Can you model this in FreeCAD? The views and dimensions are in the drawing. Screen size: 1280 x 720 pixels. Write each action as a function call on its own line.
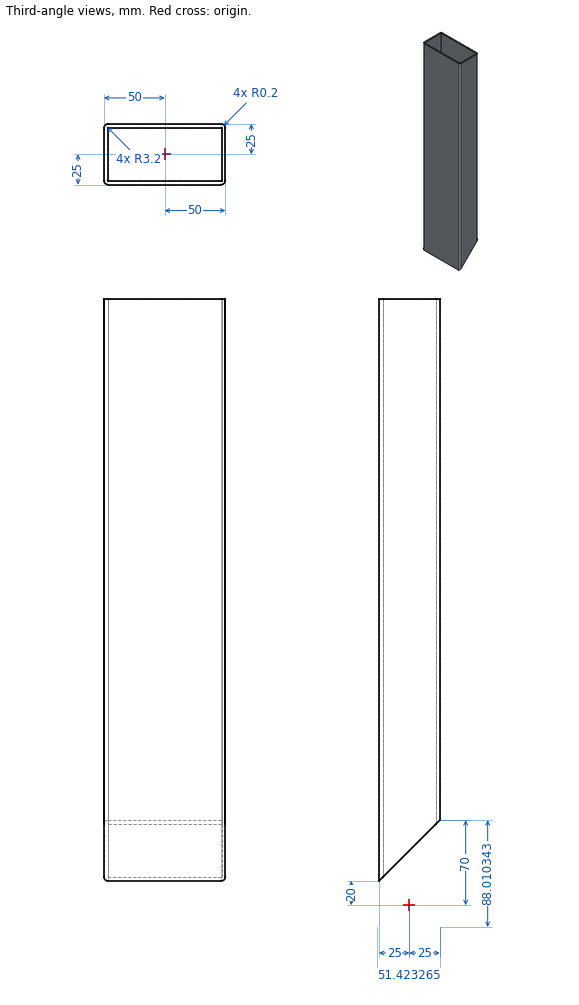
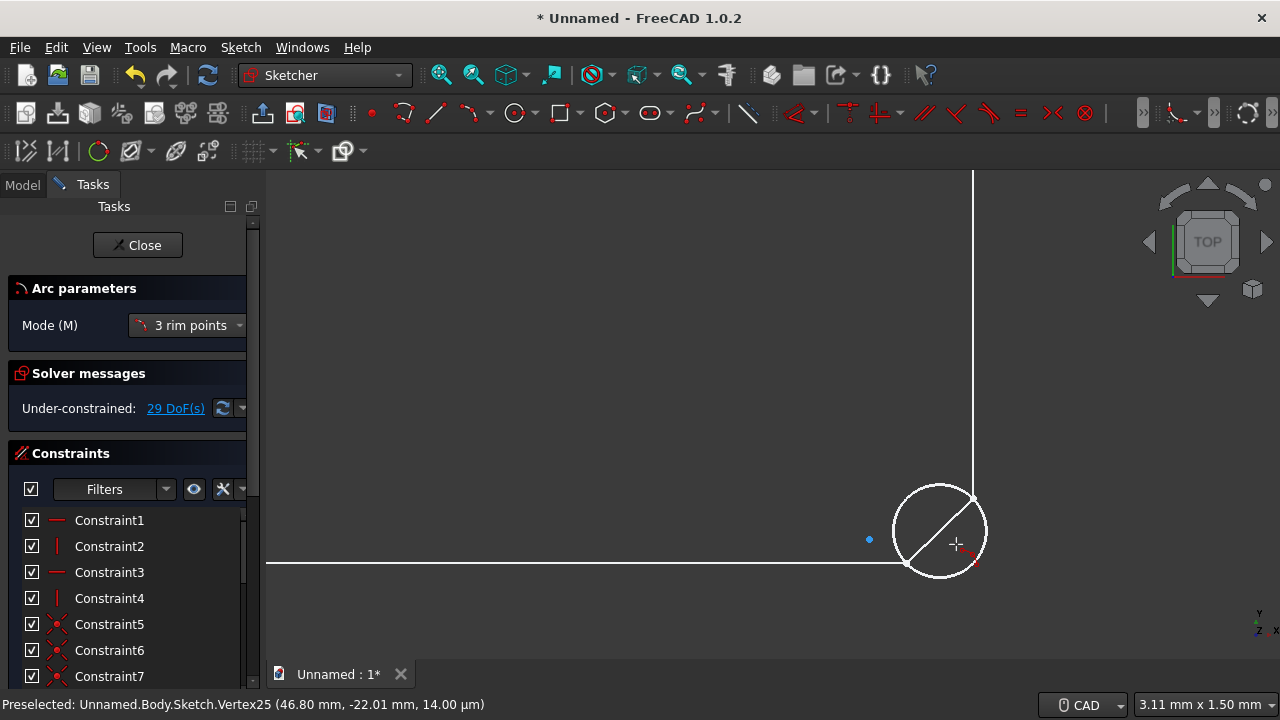
click(953, 540)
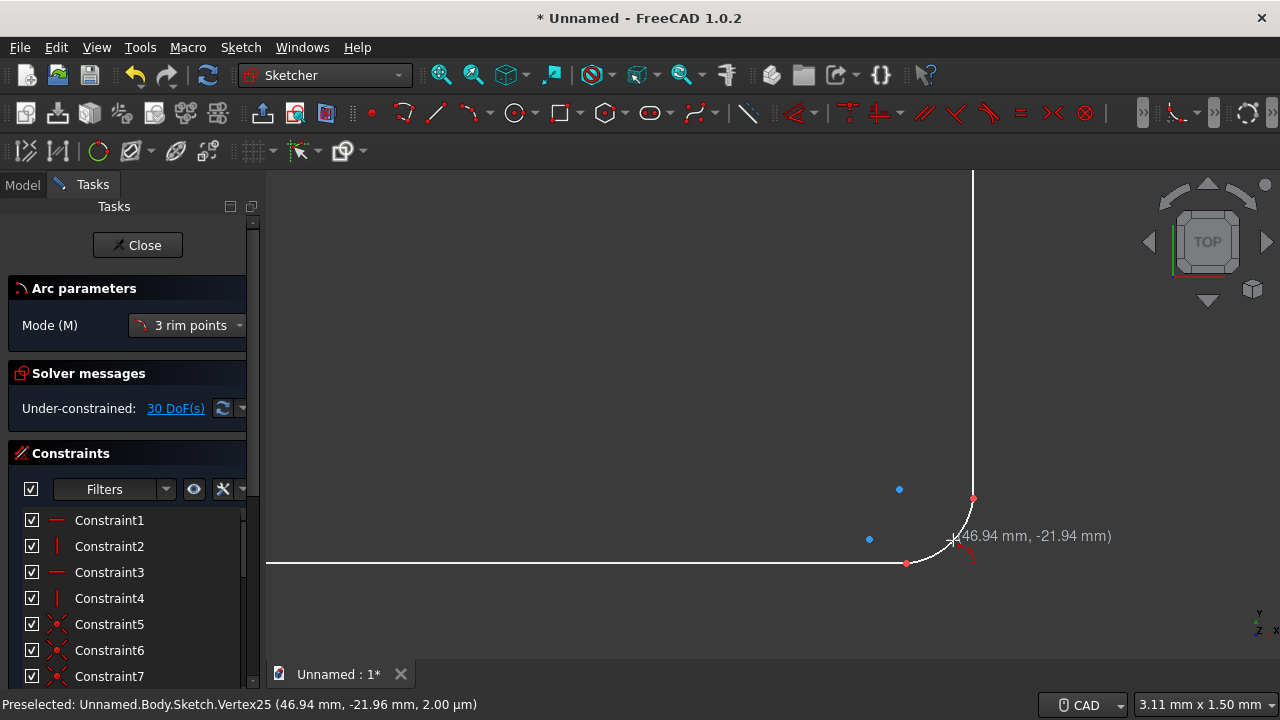
scroll(704, 414, down, 15)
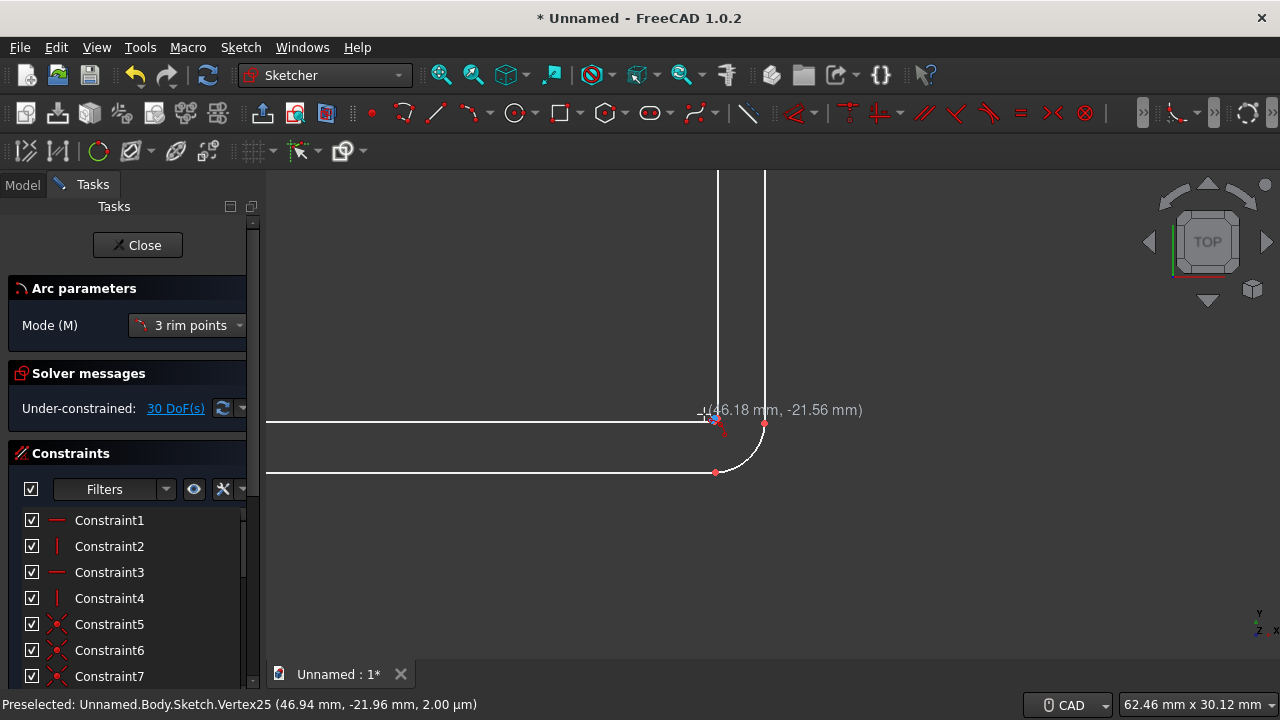
scroll(1115, 618, down, 5)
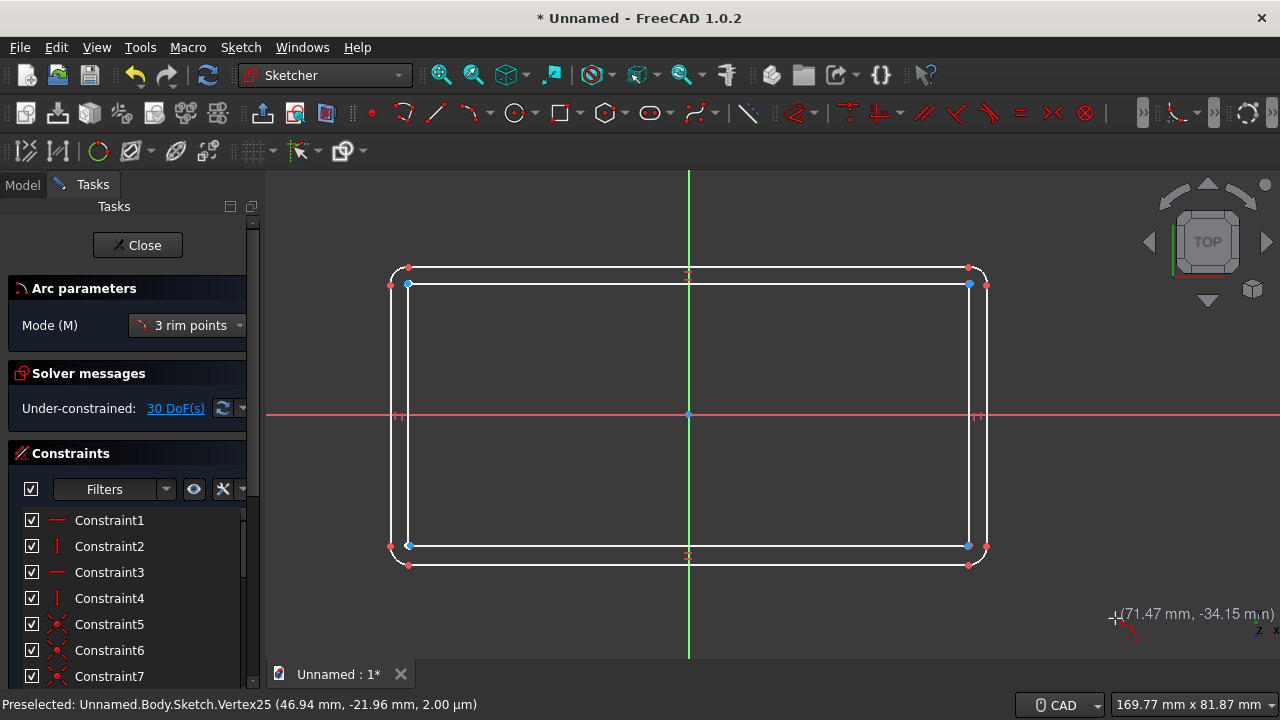
scroll(409, 546, up, 13)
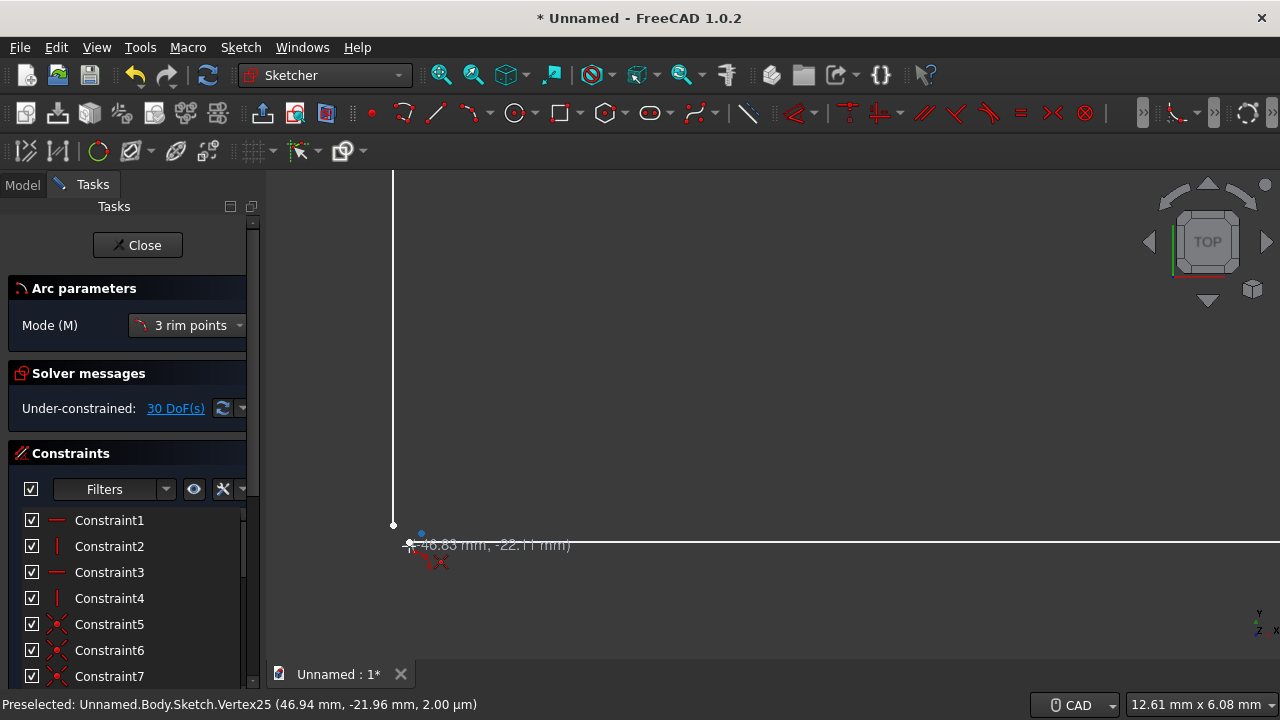
click(409, 542)
click(393, 526)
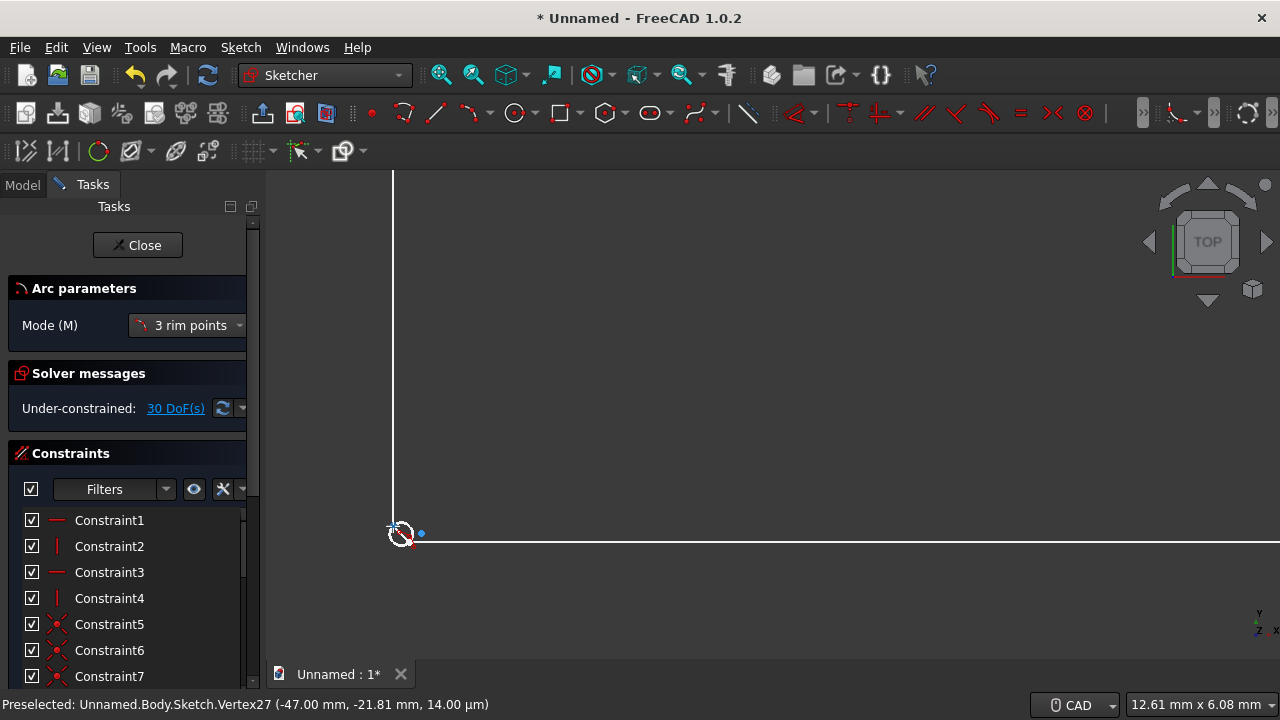
scroll(398, 537, up, 7)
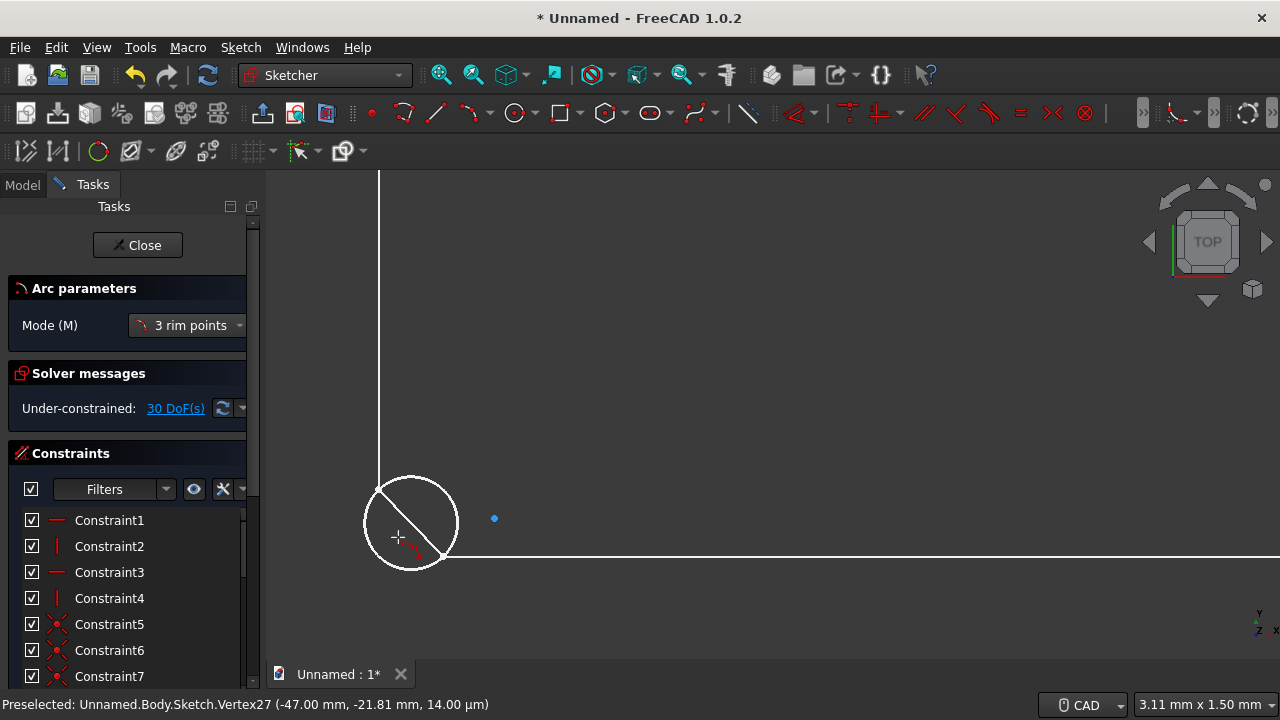
click(397, 533)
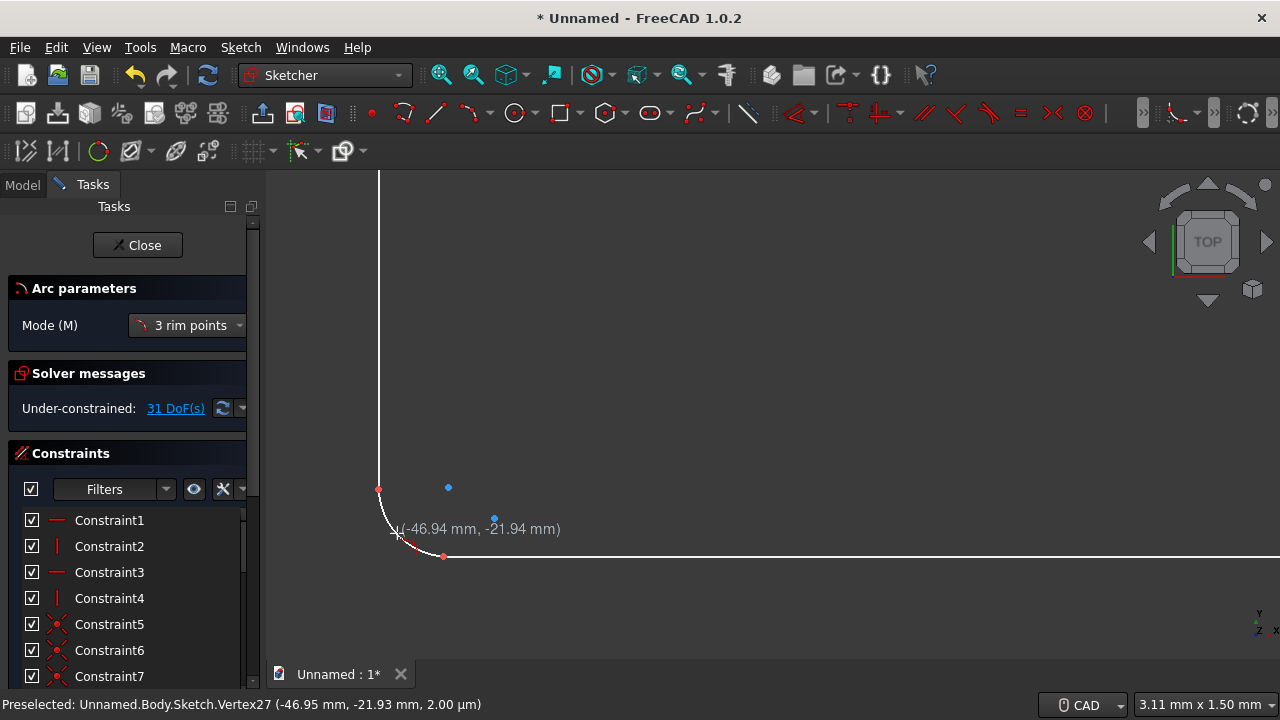
scroll(704, 414, down, 15)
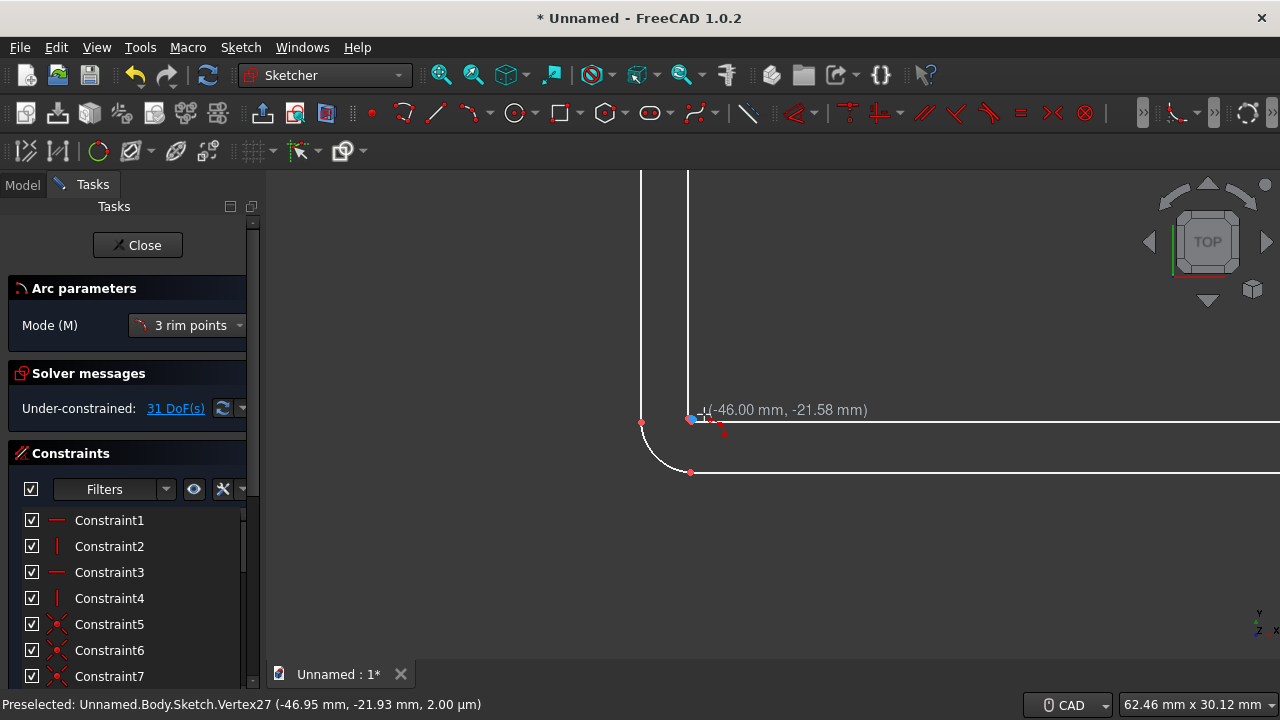
scroll(294, 618, down, 5)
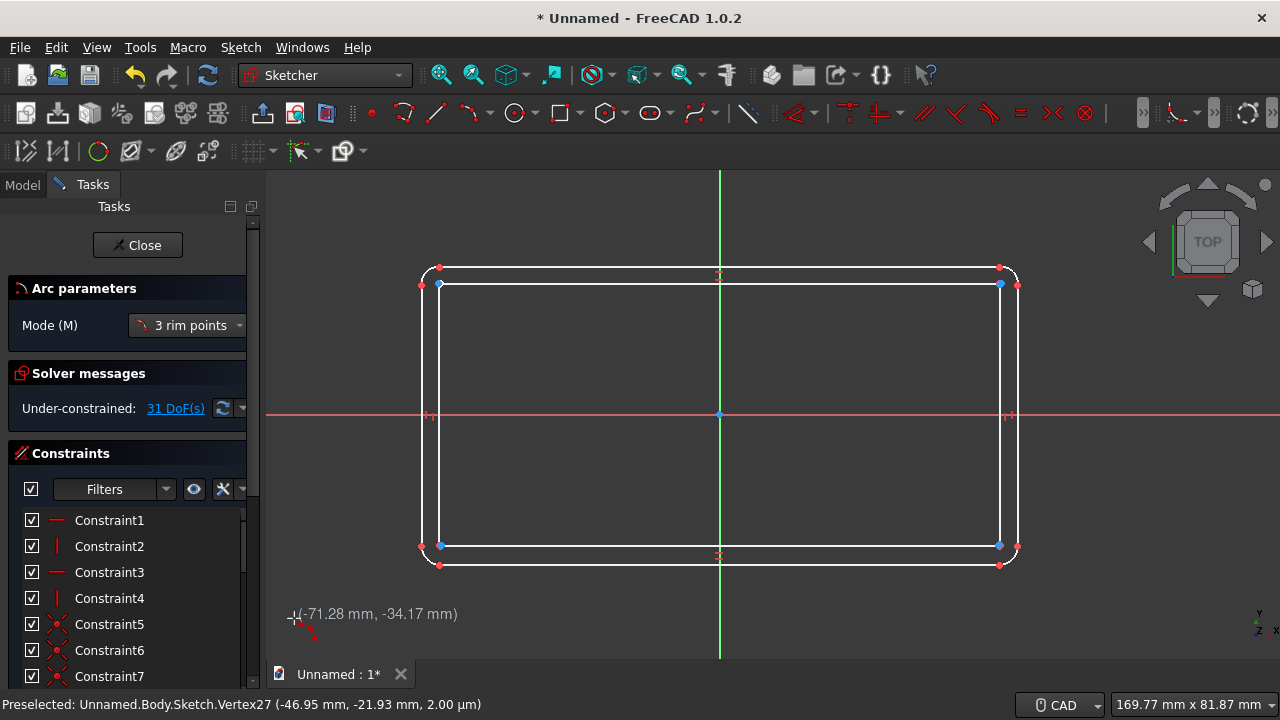
scroll(439, 285, up, 13)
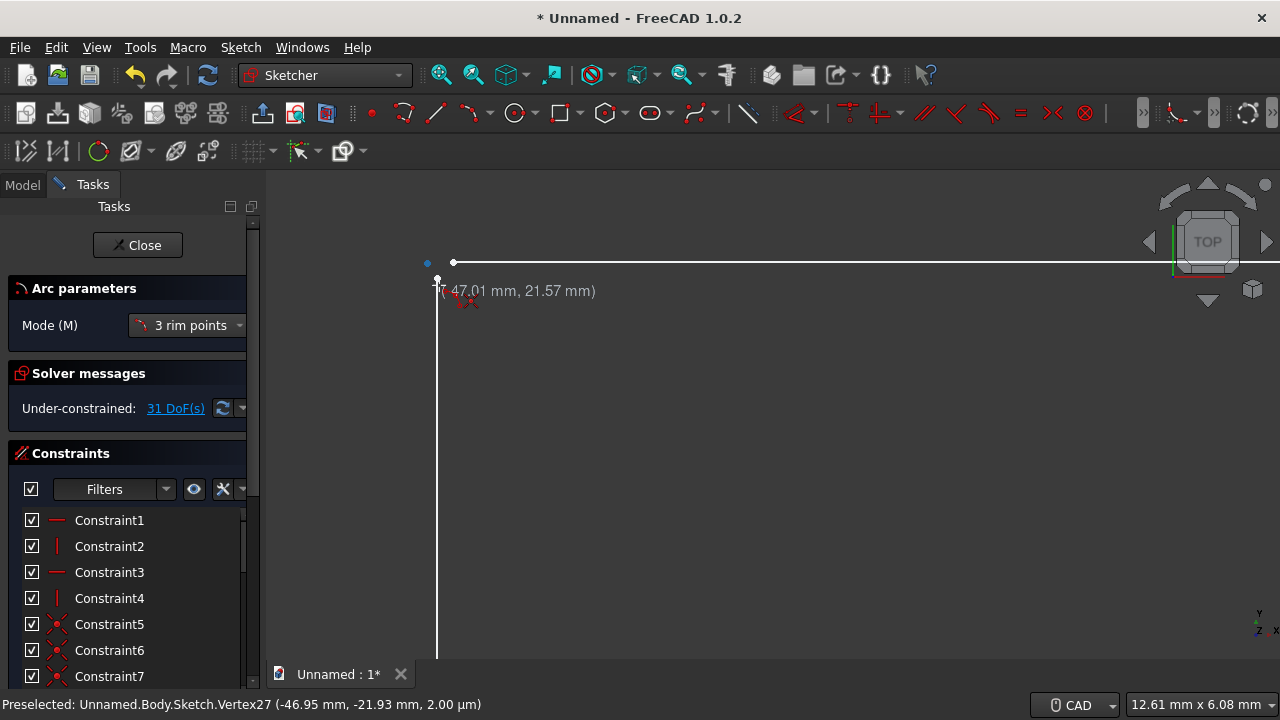
click(437, 279)
click(453, 262)